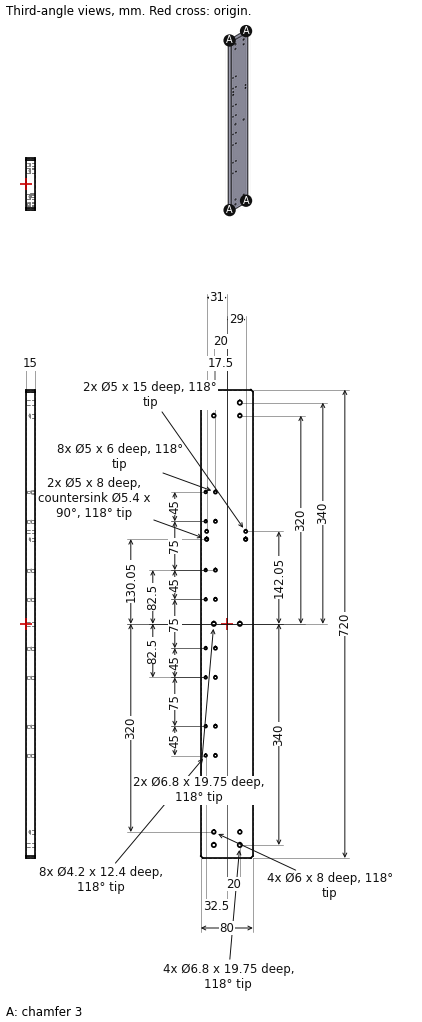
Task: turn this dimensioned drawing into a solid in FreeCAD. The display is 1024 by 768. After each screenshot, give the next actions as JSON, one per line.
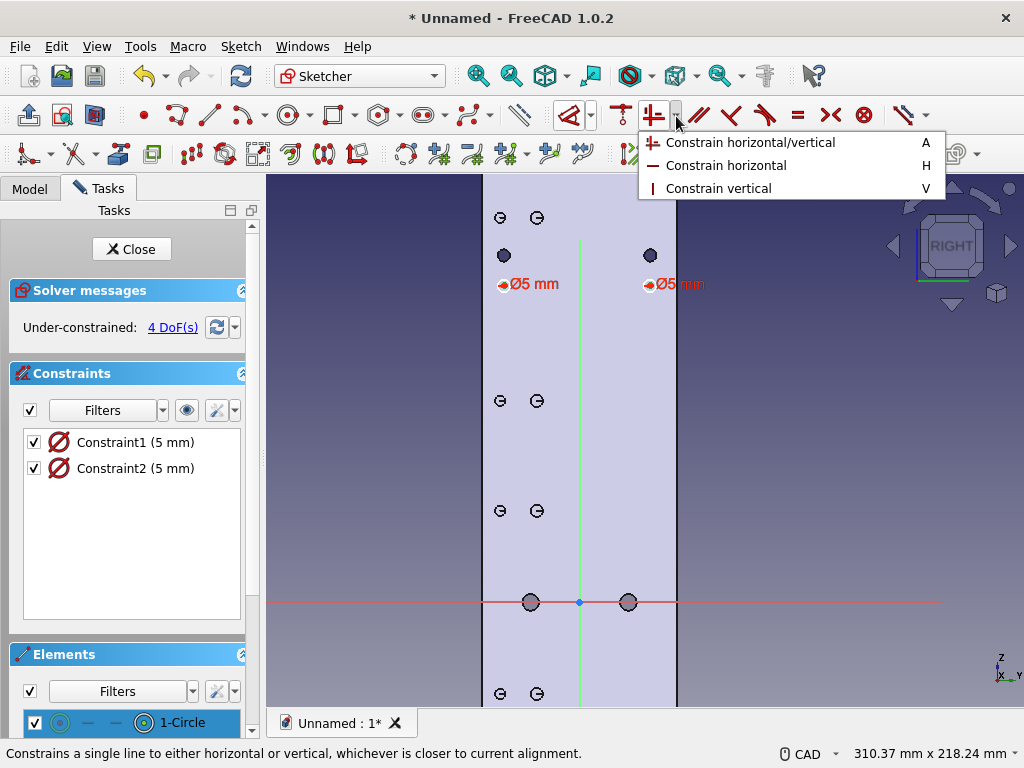
{"action": "left_click", "coordinate": [792, 166]}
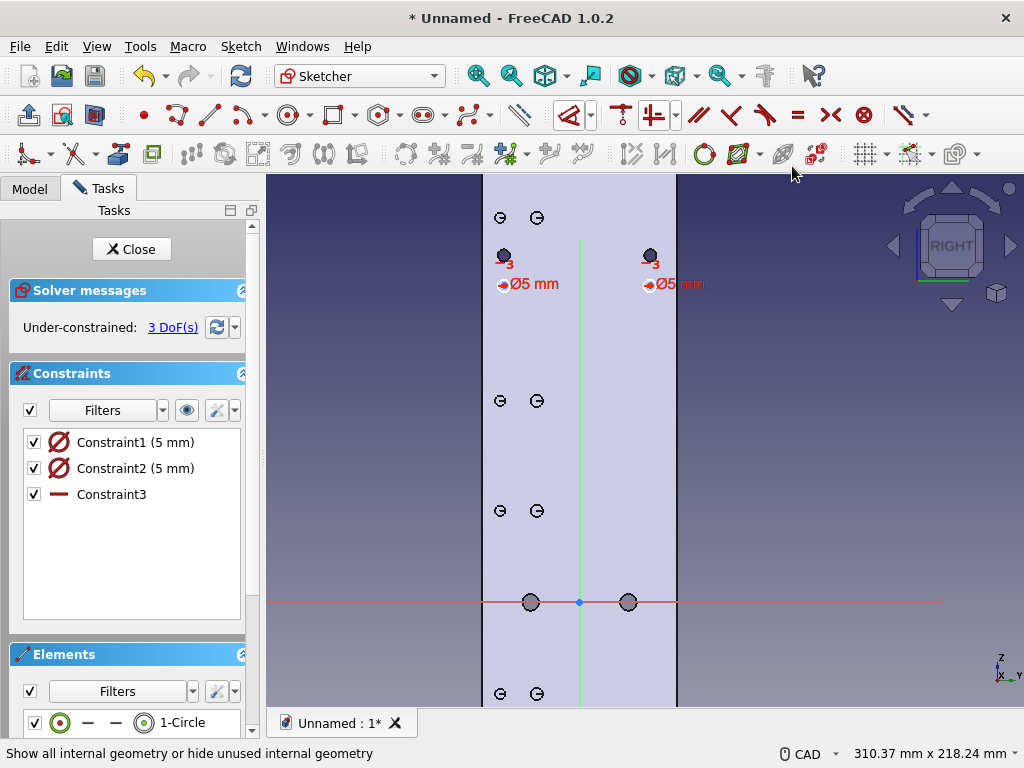
{"action": "left_click", "coordinate": [504, 286]}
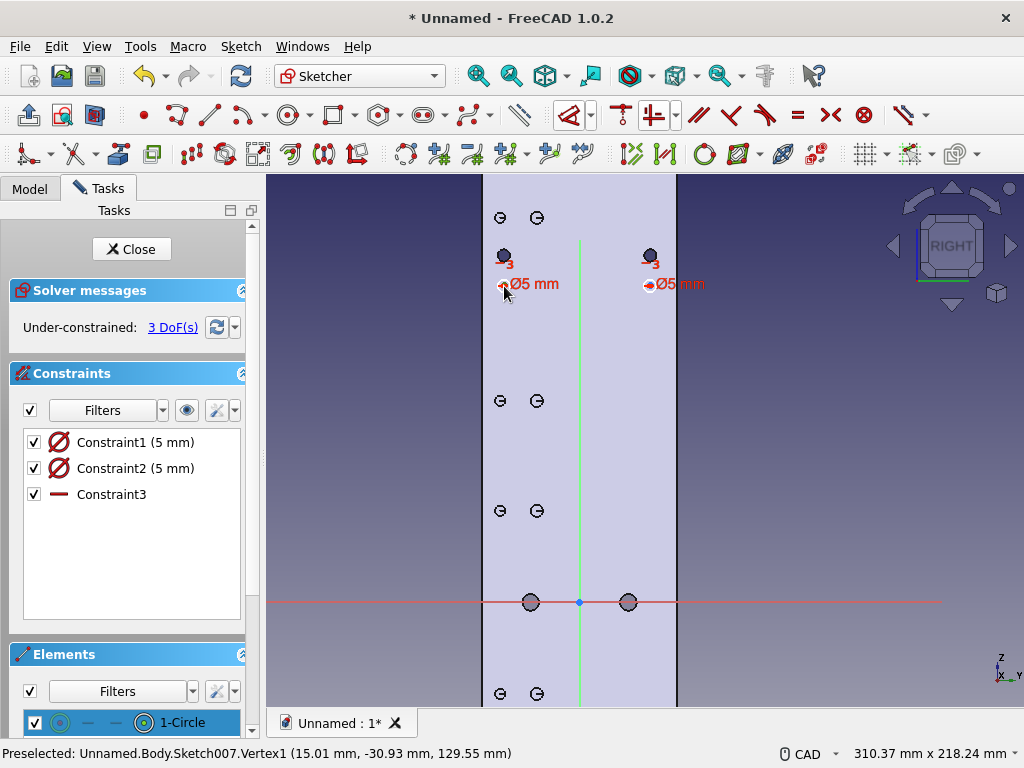
{"action": "key", "text": "l"}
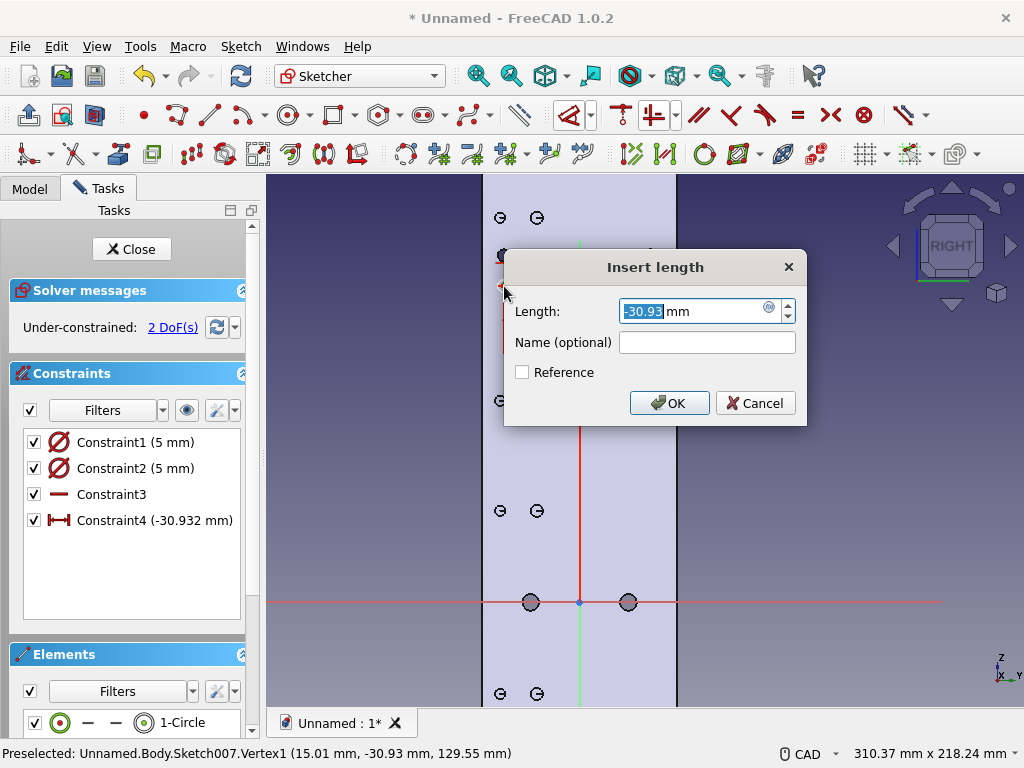
{"action": "type", "text": "-31"}
{"action": "key", "text": "Return"}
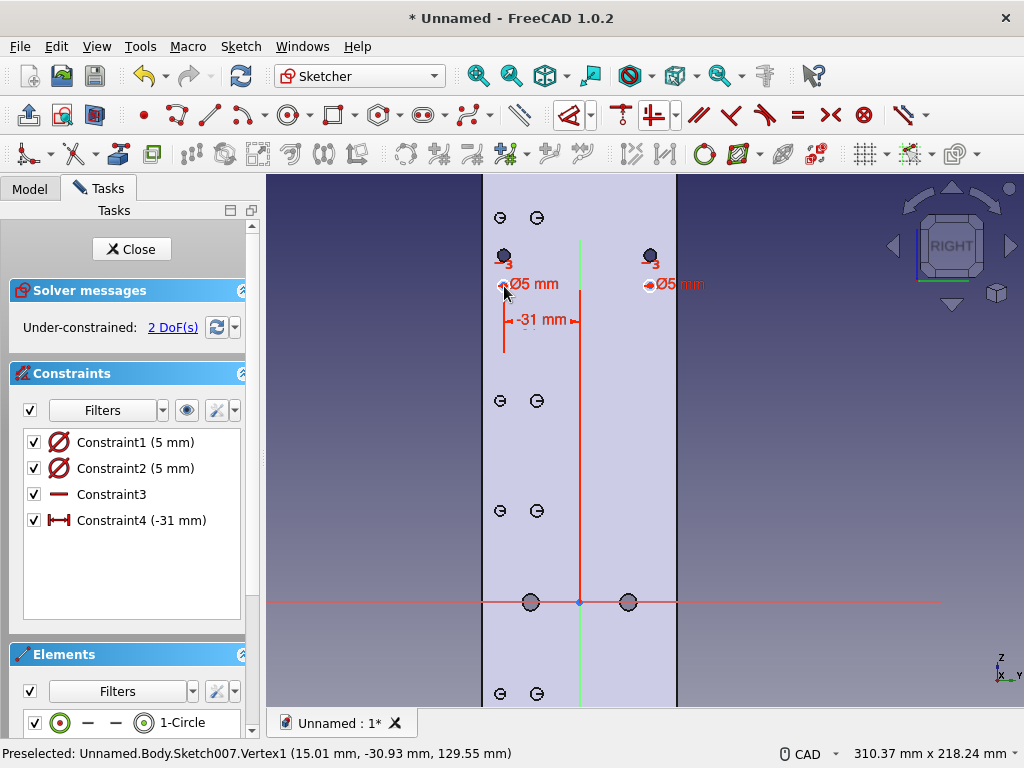
{"action": "left_click", "coordinate": [650, 286]}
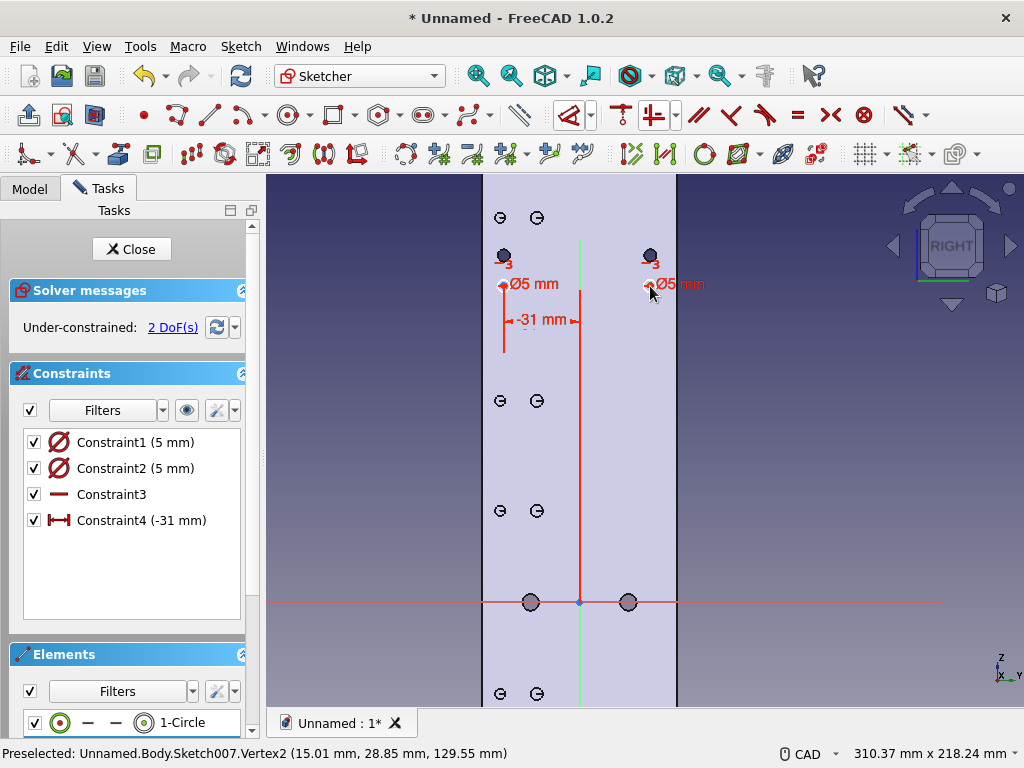
{"action": "key", "text": "l"}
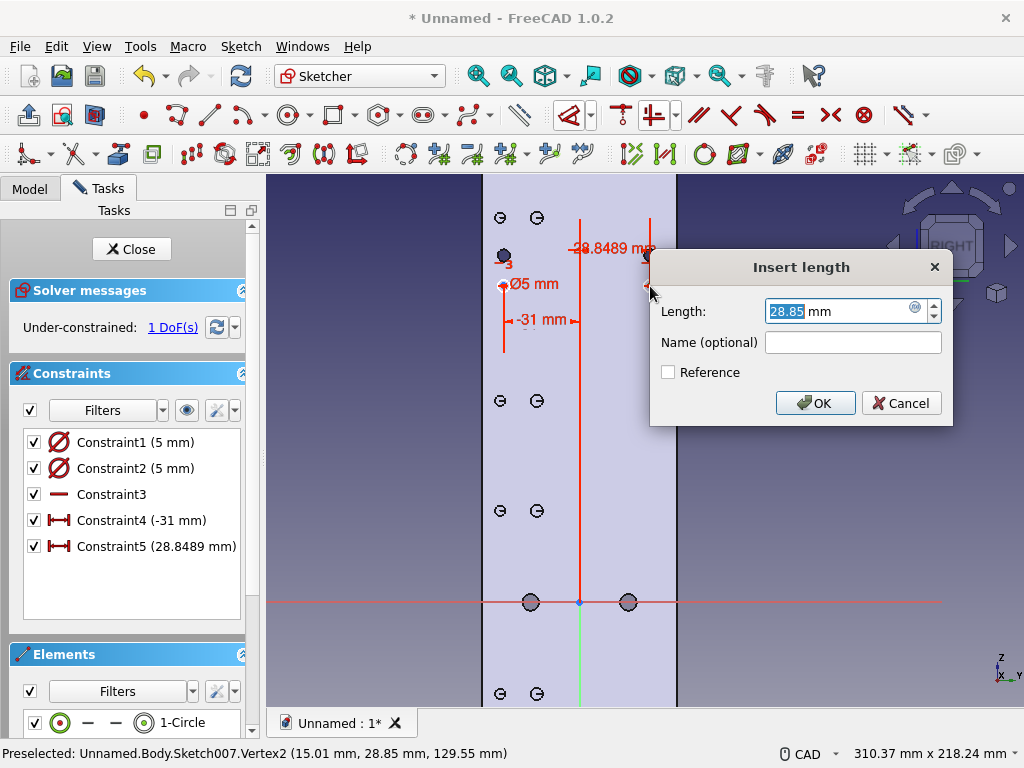
{"action": "type", "text": "29"}
{"action": "key", "text": "Return"}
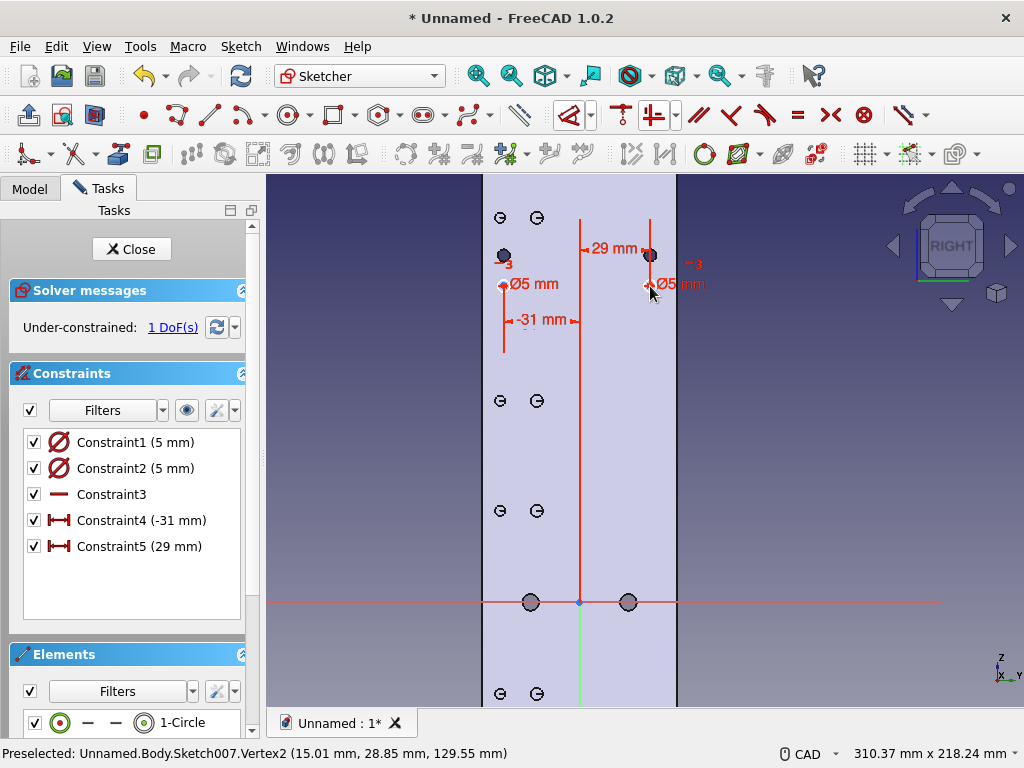
{"action": "left_click", "coordinate": [504, 286]}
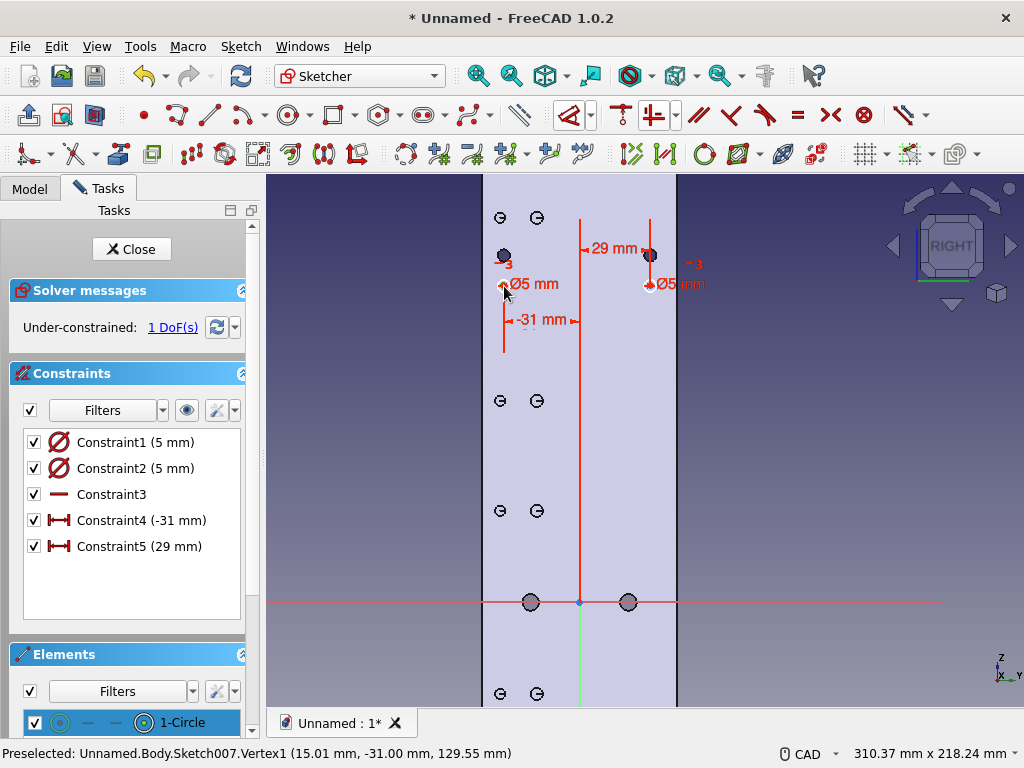
{"action": "key", "text": "i"}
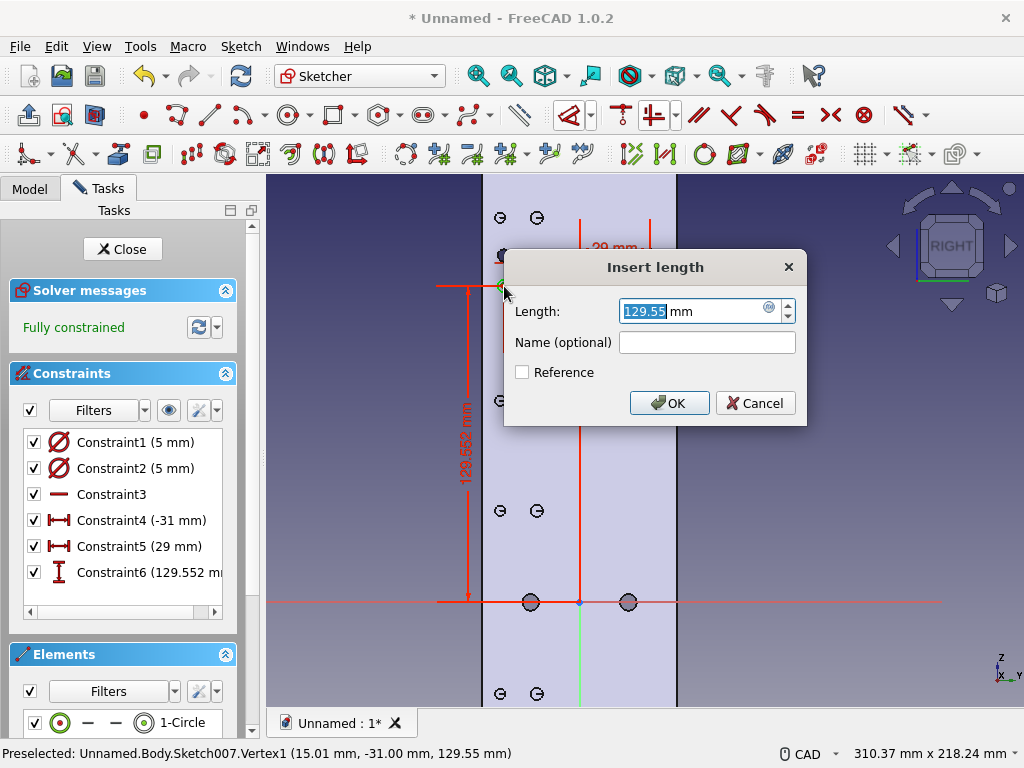
{"action": "type", "text": "130.05"}
{"action": "key", "text": "Return"}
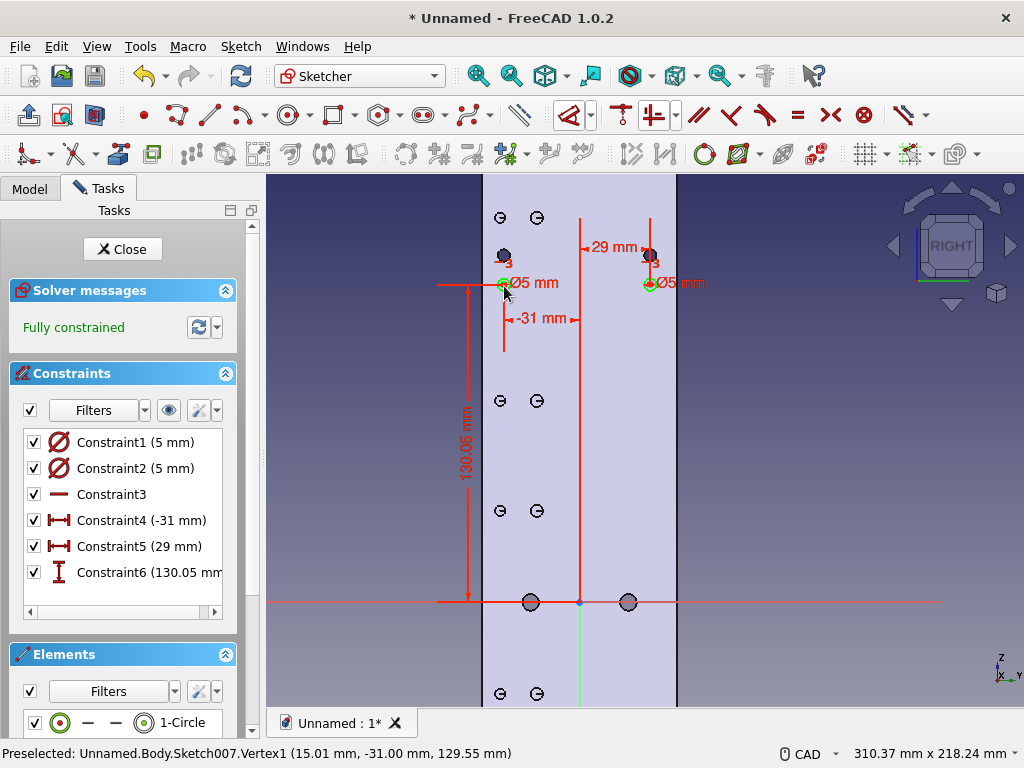
{"action": "left_click", "coordinate": [123, 249]}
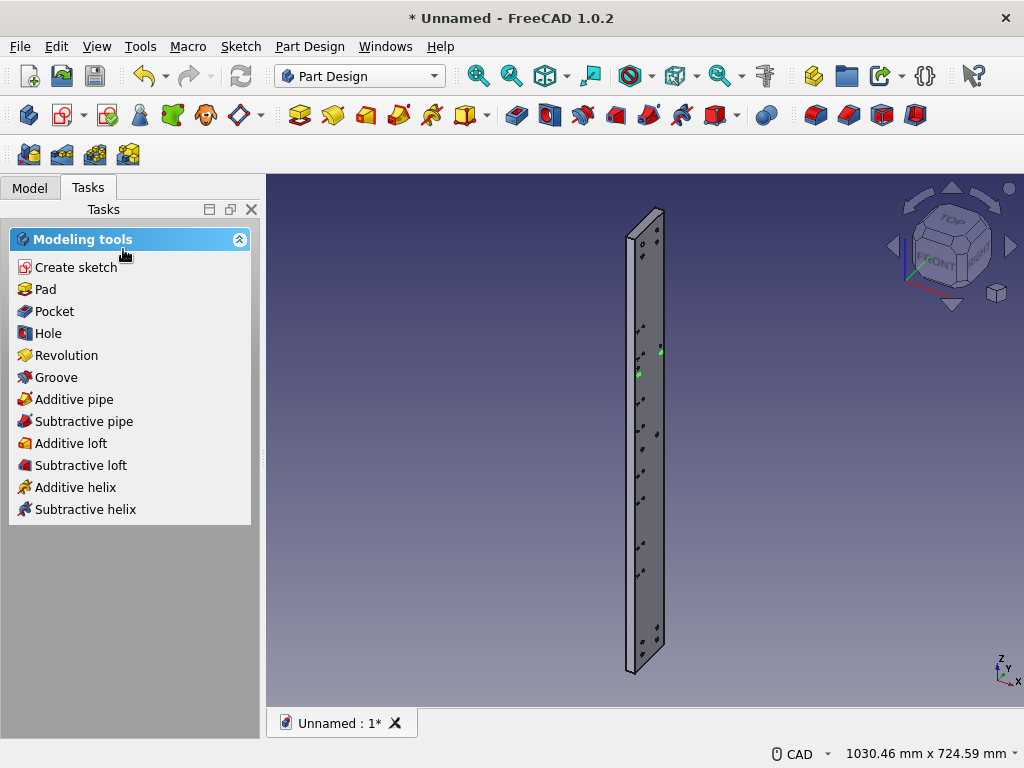
{"action": "left_click", "coordinate": [550, 116]}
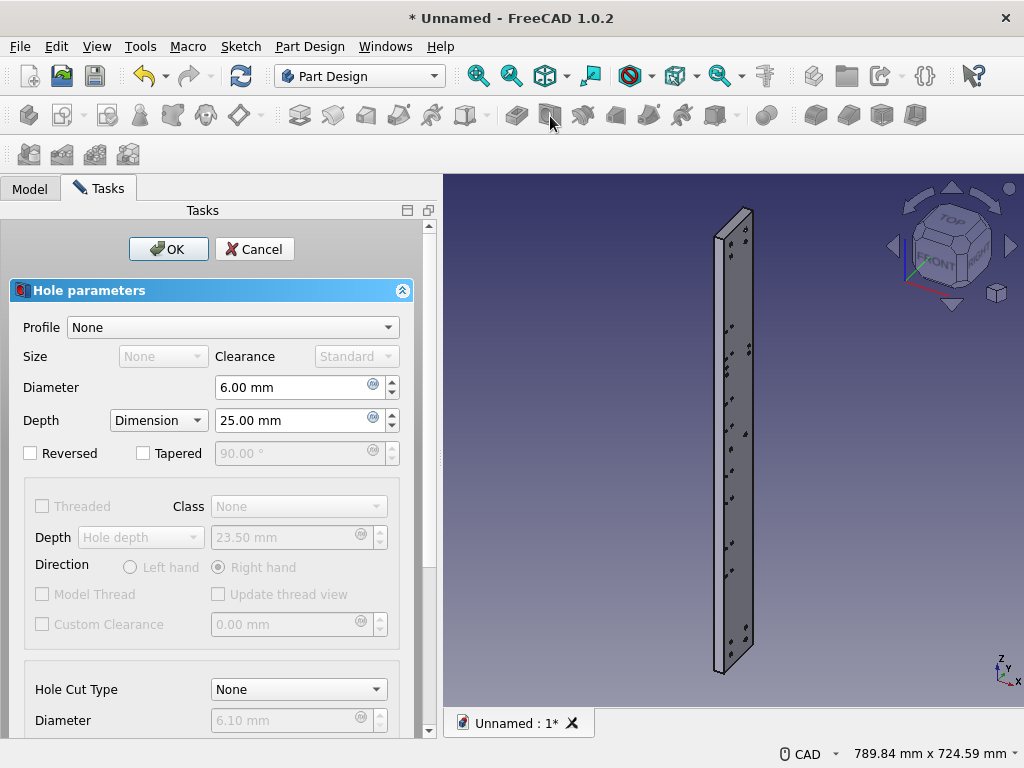
{"action": "triple_click", "coordinate": [300, 388]}